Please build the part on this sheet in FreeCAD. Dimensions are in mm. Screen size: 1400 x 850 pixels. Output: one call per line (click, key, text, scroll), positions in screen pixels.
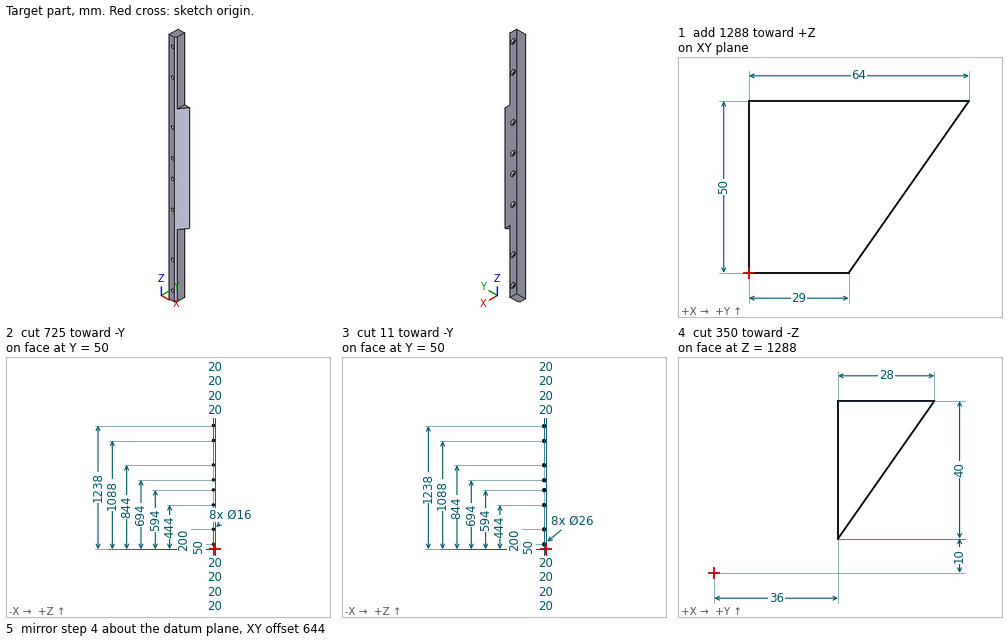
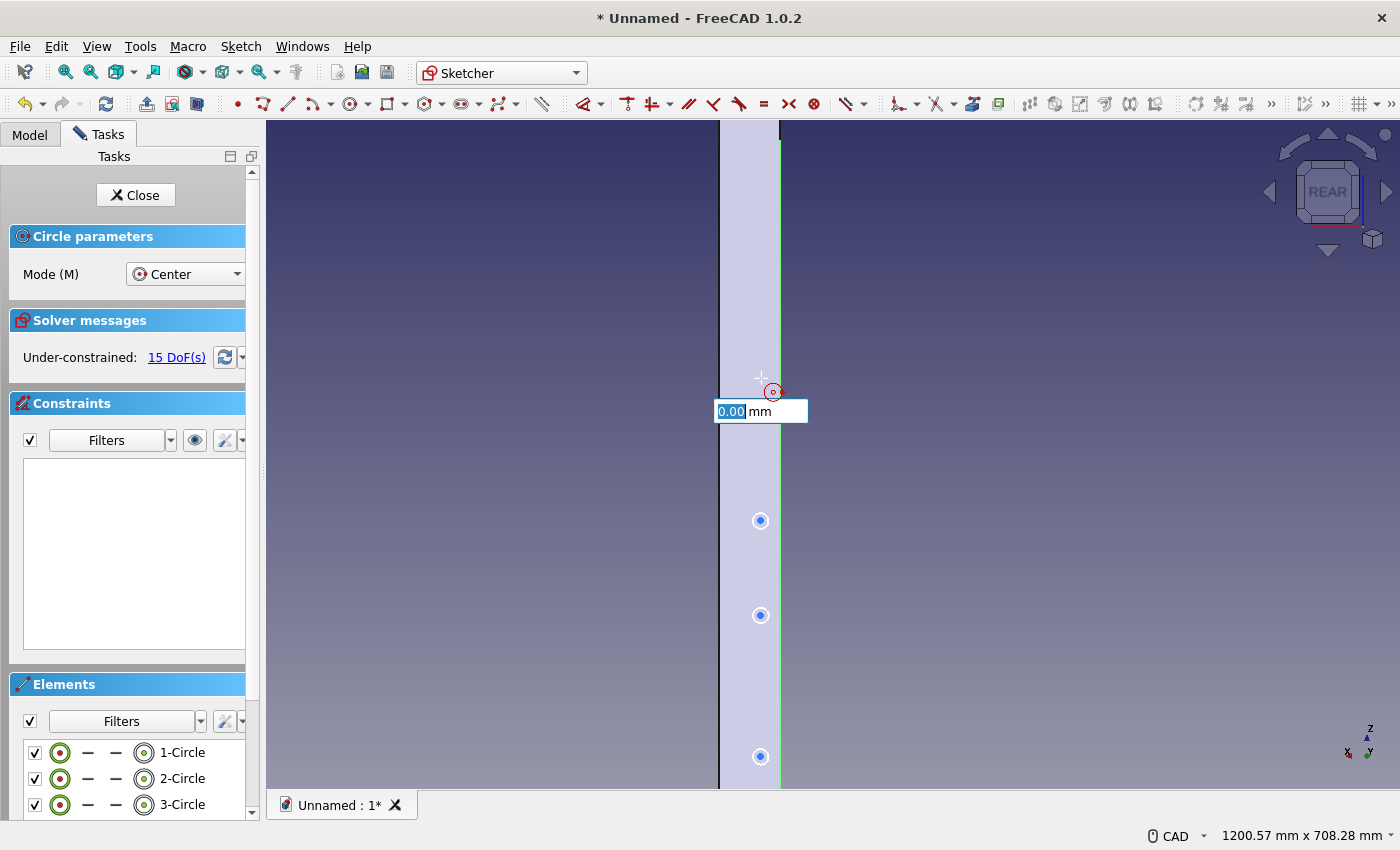
scroll(756, 373, up, 4)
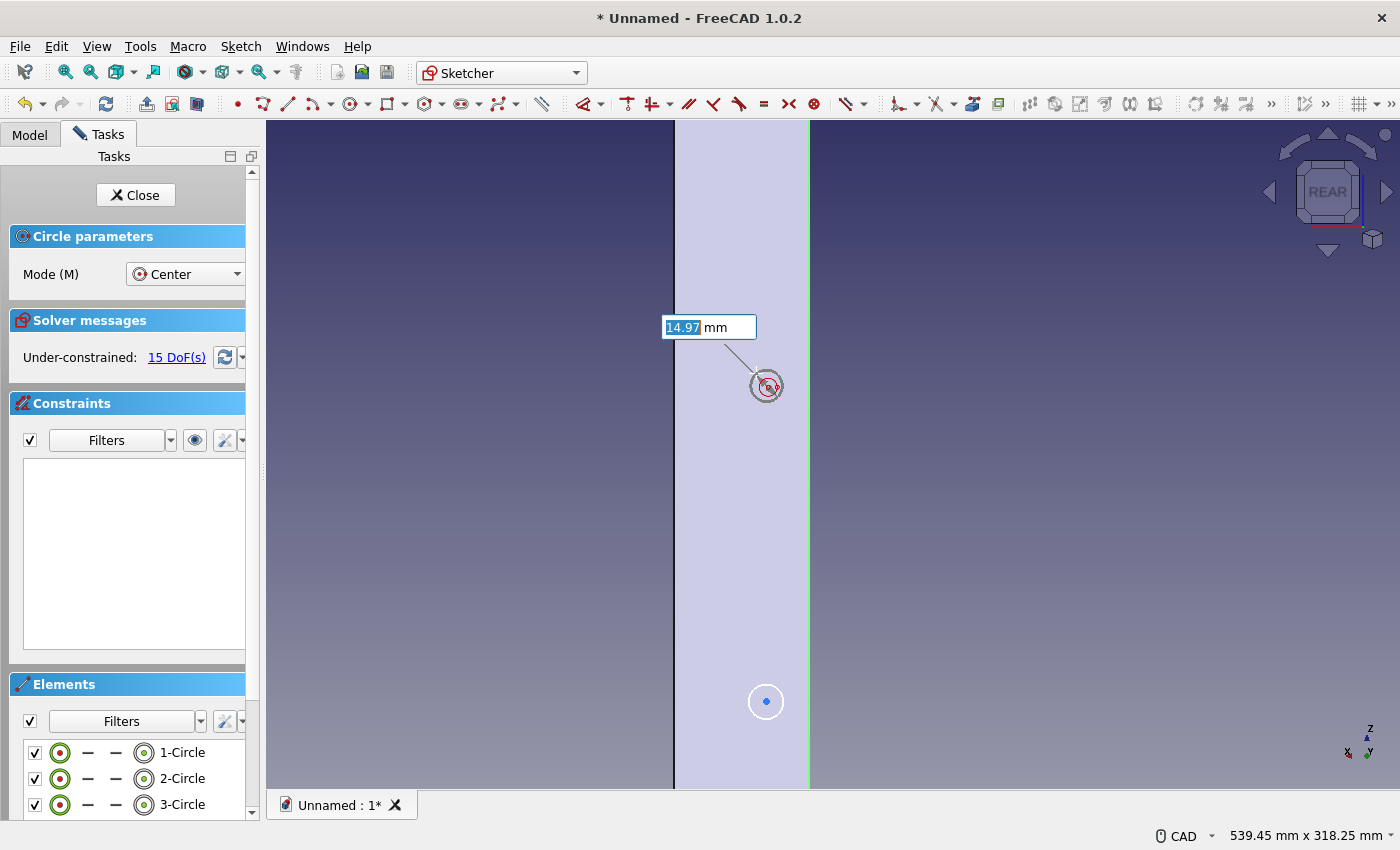
click(755, 373)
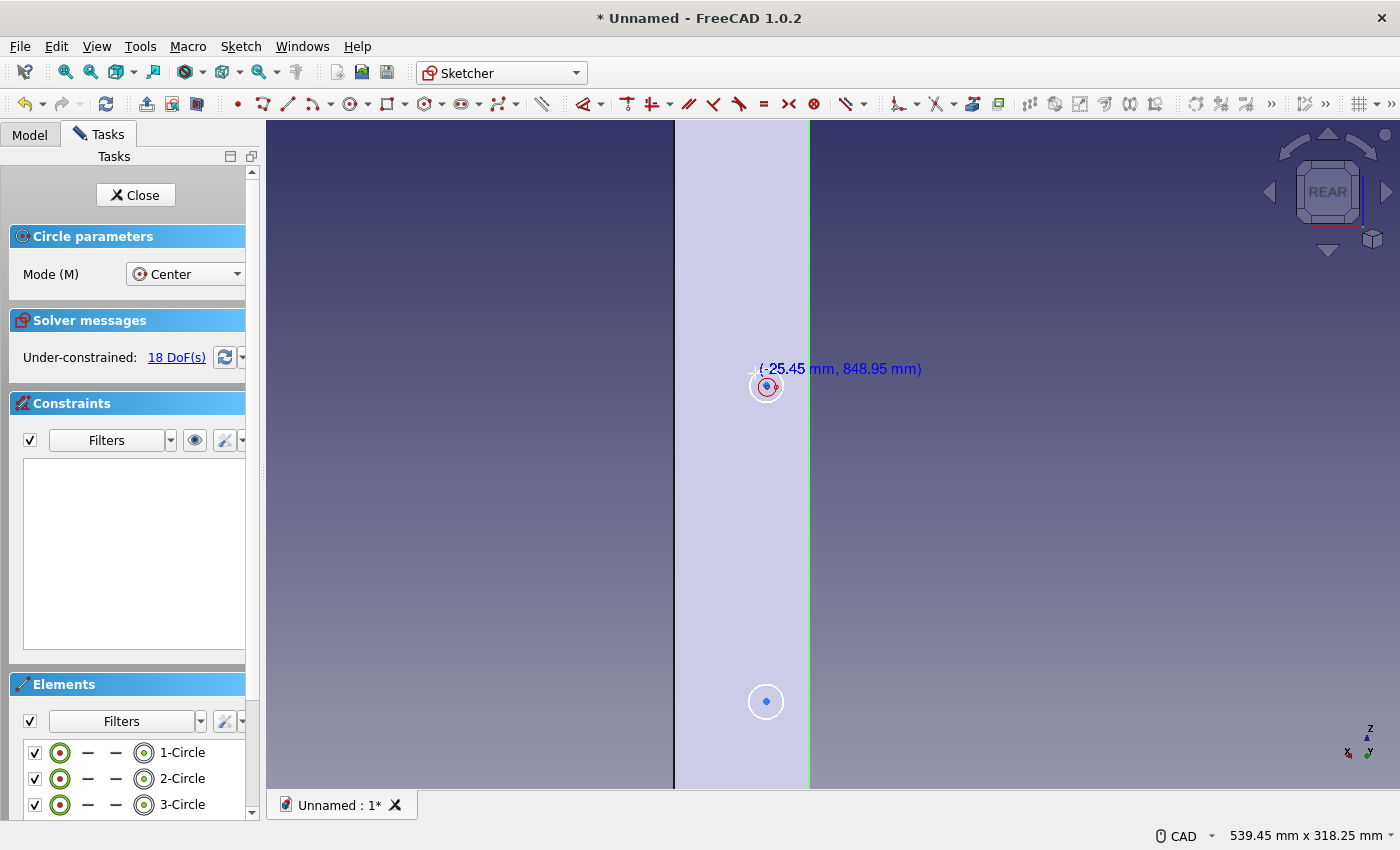
scroll(762, 376, down, 9)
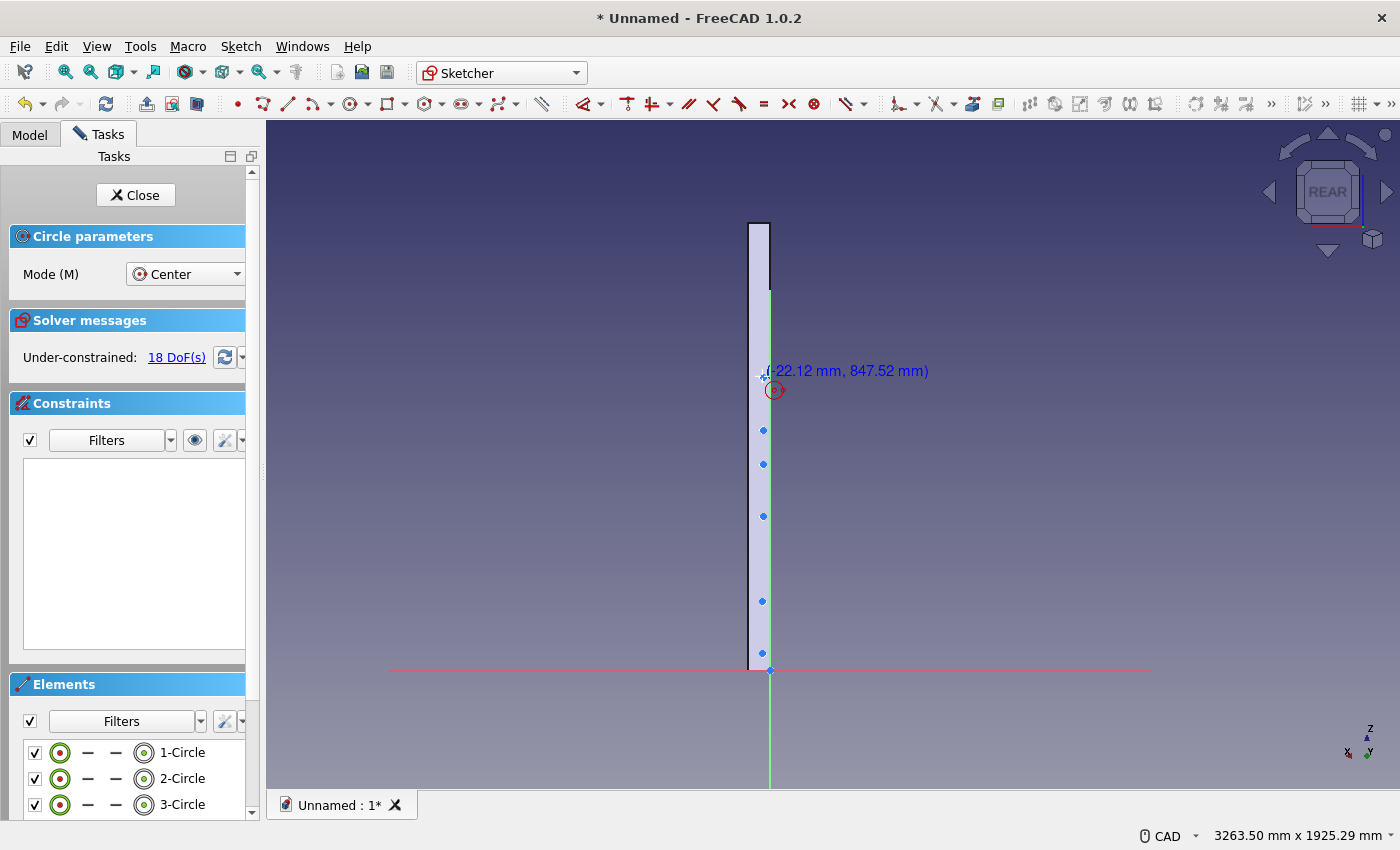
scroll(763, 293, up, 11)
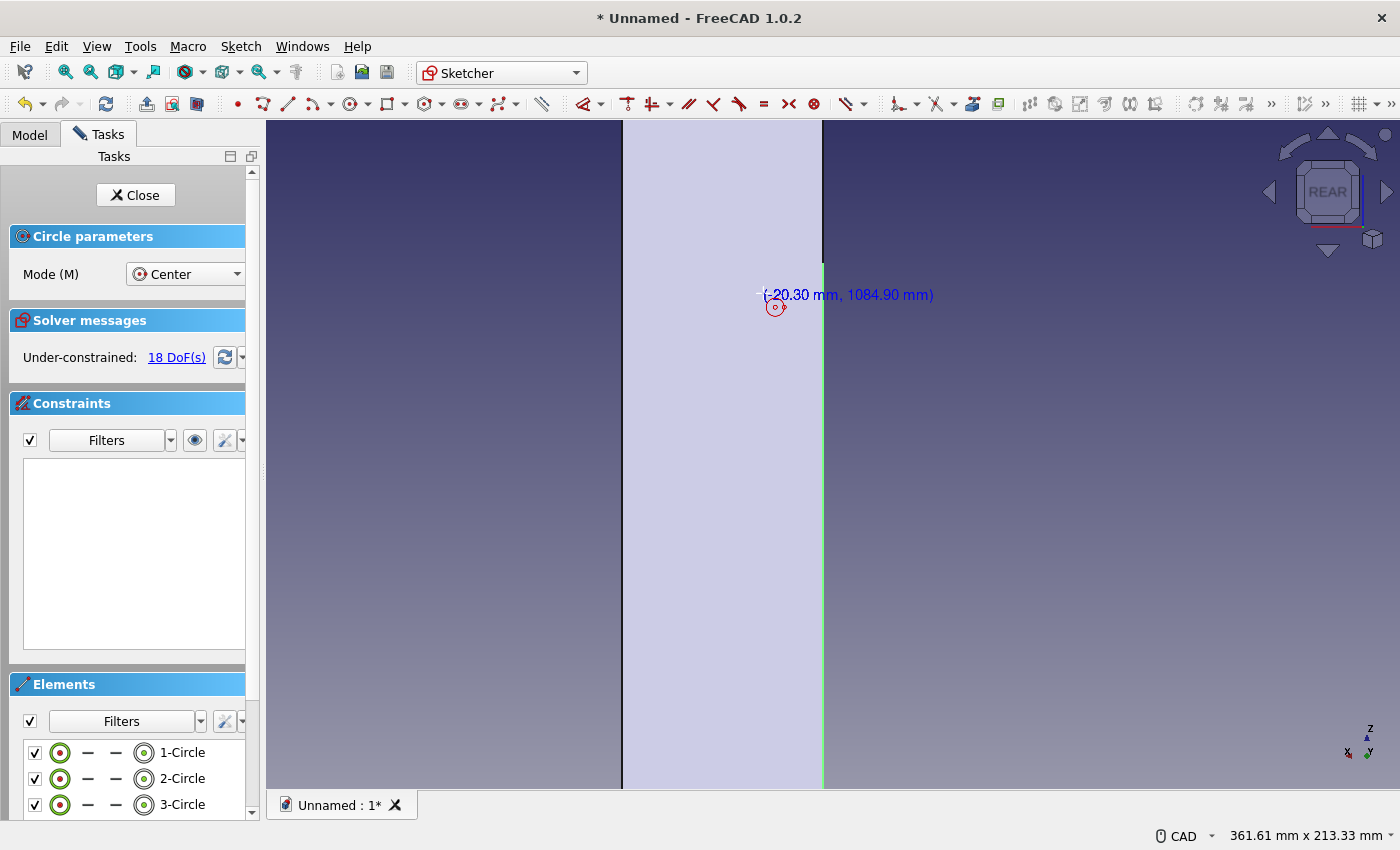
scroll(763, 293, down, 11)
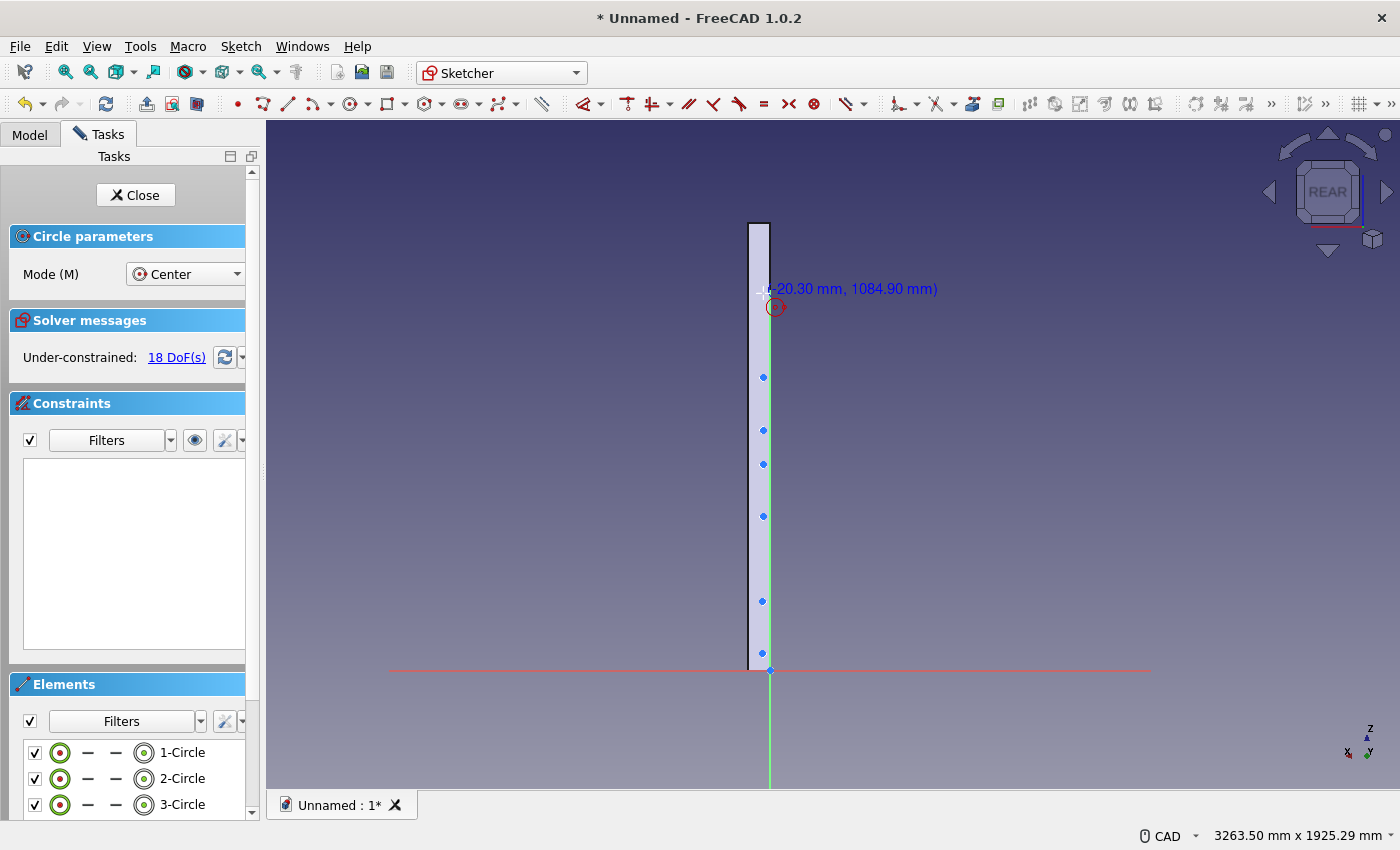
scroll(763, 293, up, 5)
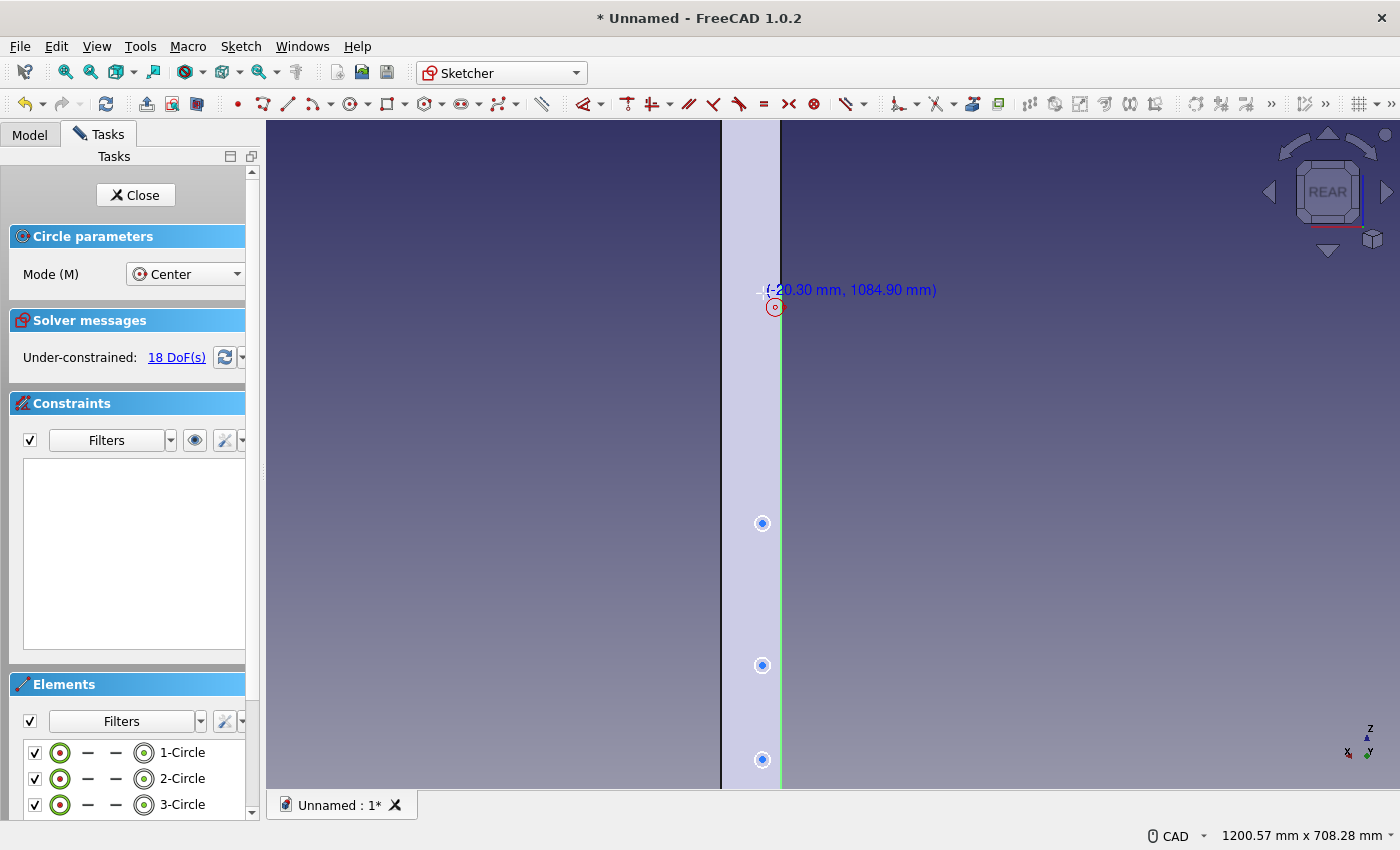
click(763, 292)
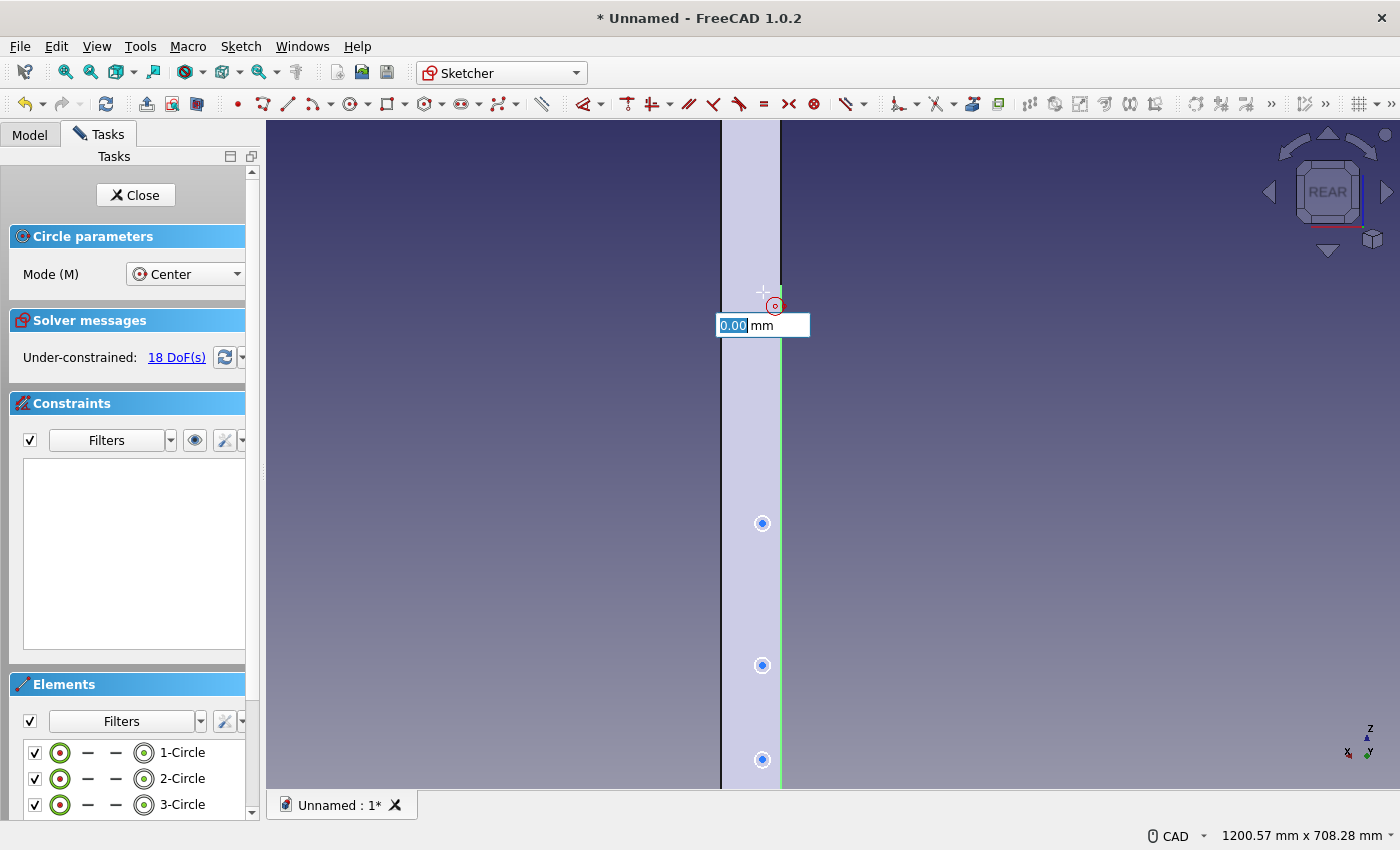
scroll(757, 287, up, 4)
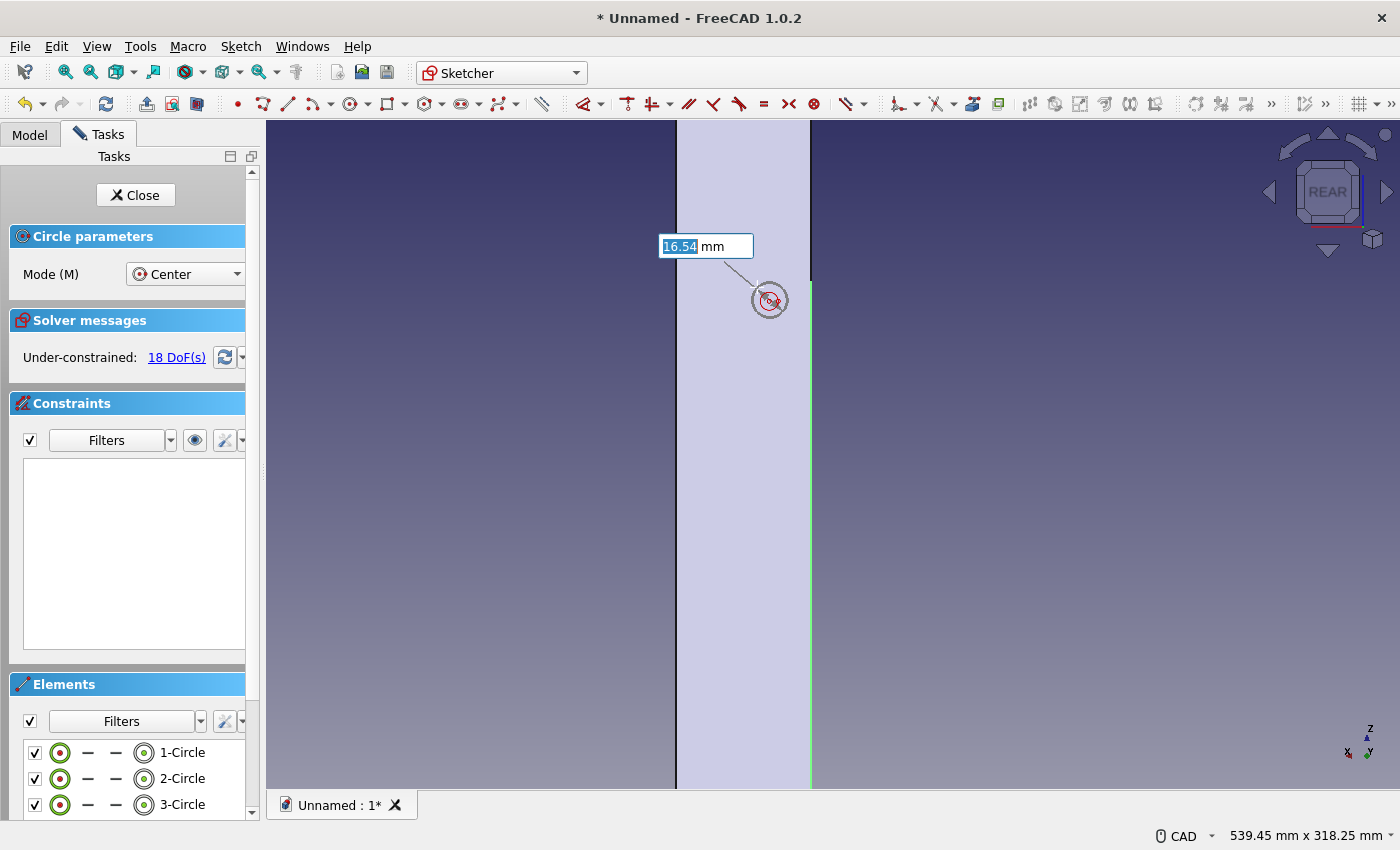
click(757, 287)